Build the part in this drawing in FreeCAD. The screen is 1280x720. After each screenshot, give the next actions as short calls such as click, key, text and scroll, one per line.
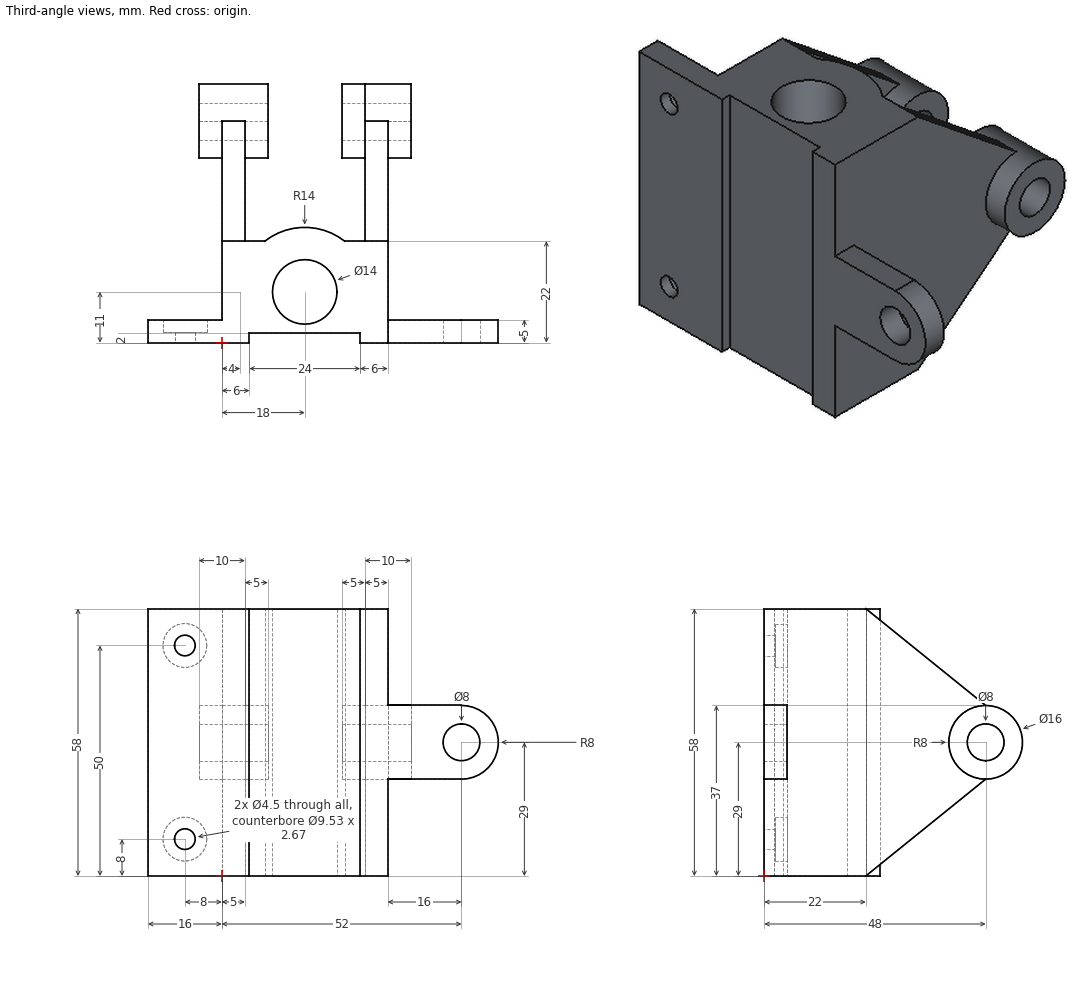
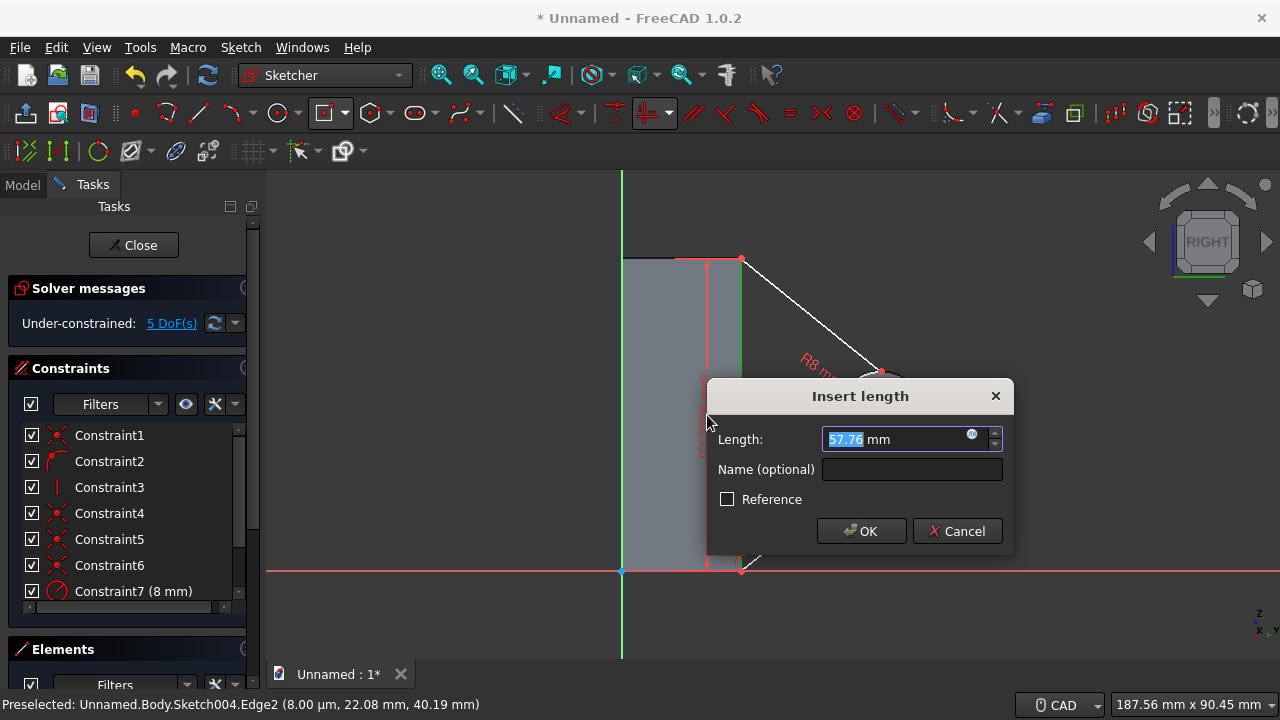
text(58)
key(Return)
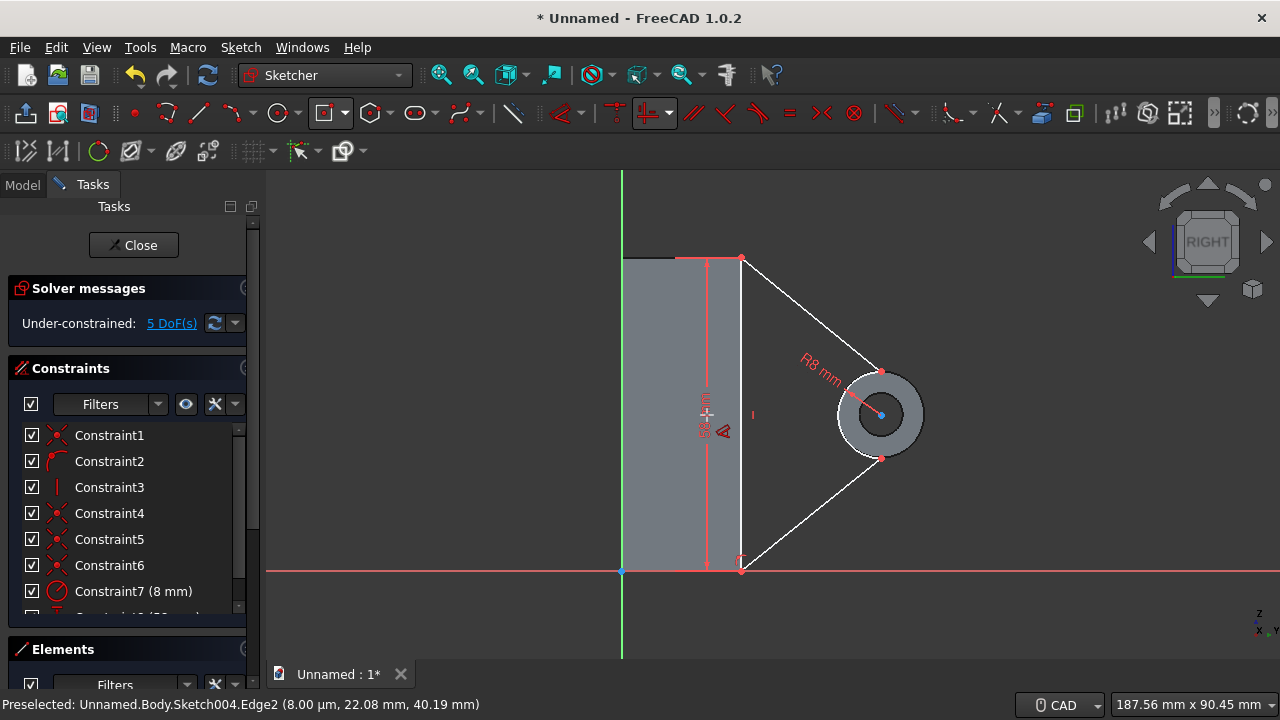
click(881, 372)
click(751, 605)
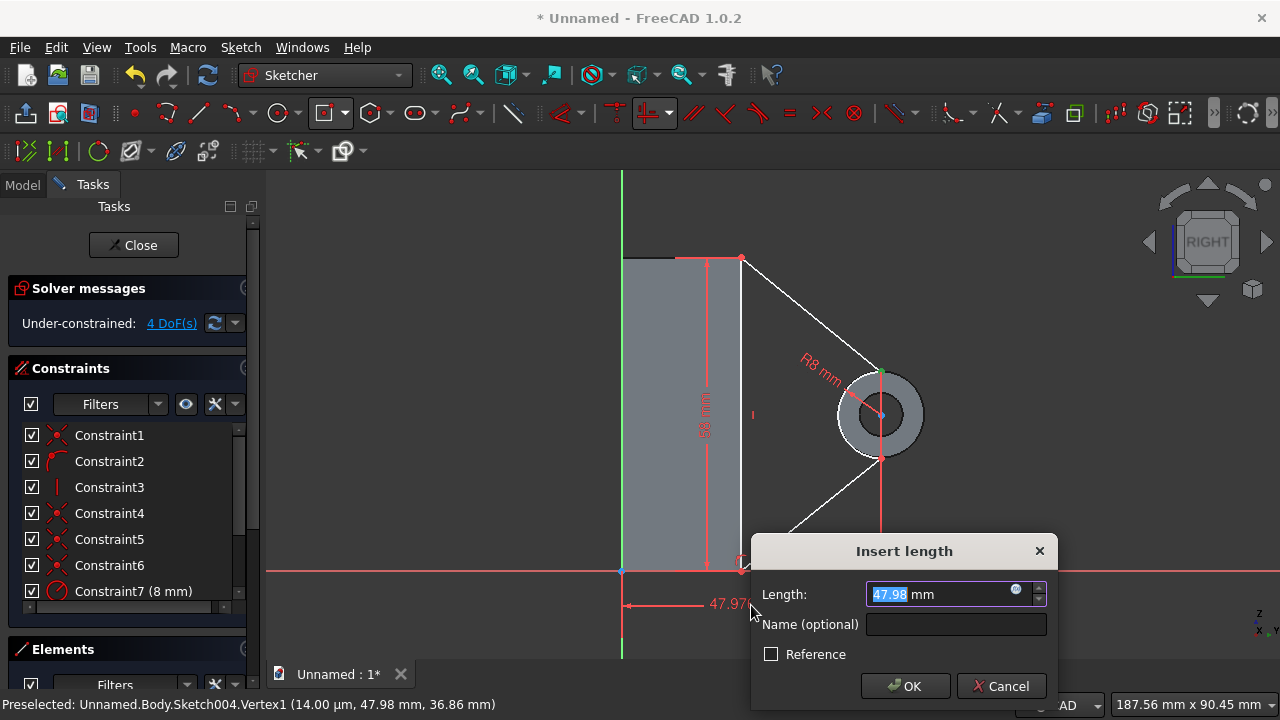
text(48)
key(Return)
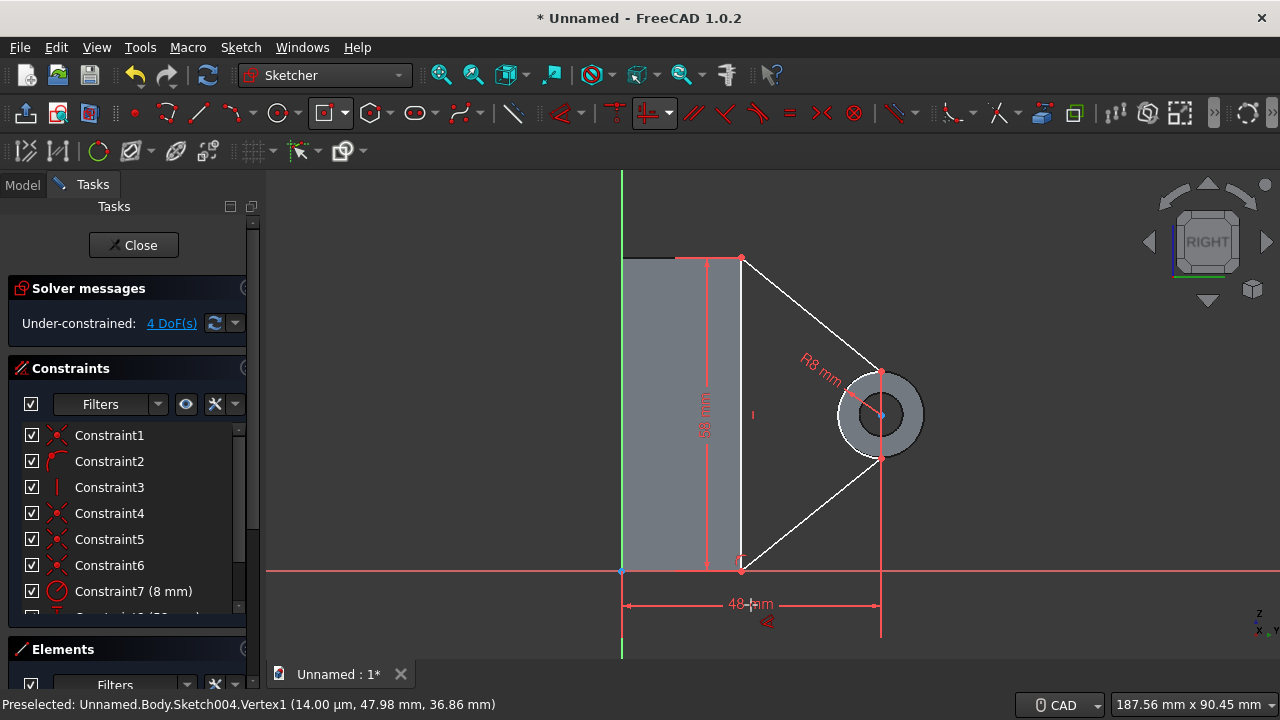
click(881, 372)
click(915, 472)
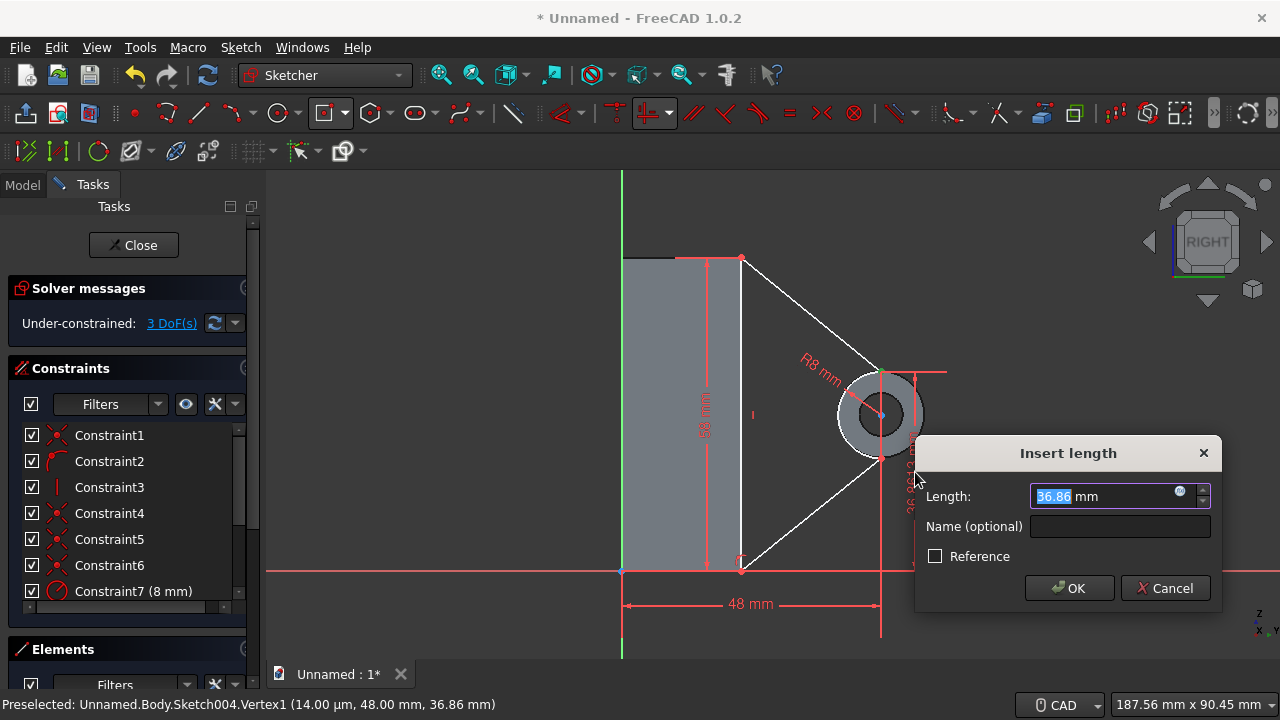
text(37)
key(Return)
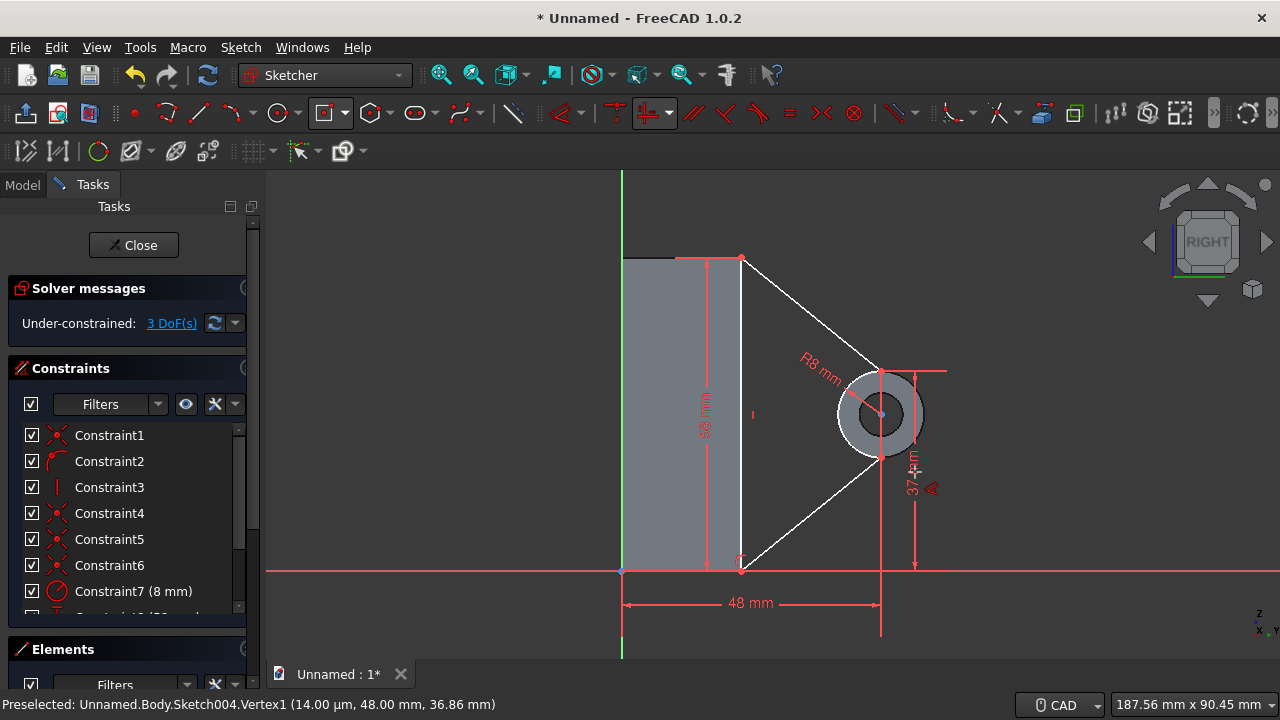
click(741, 258)
click(654, 605)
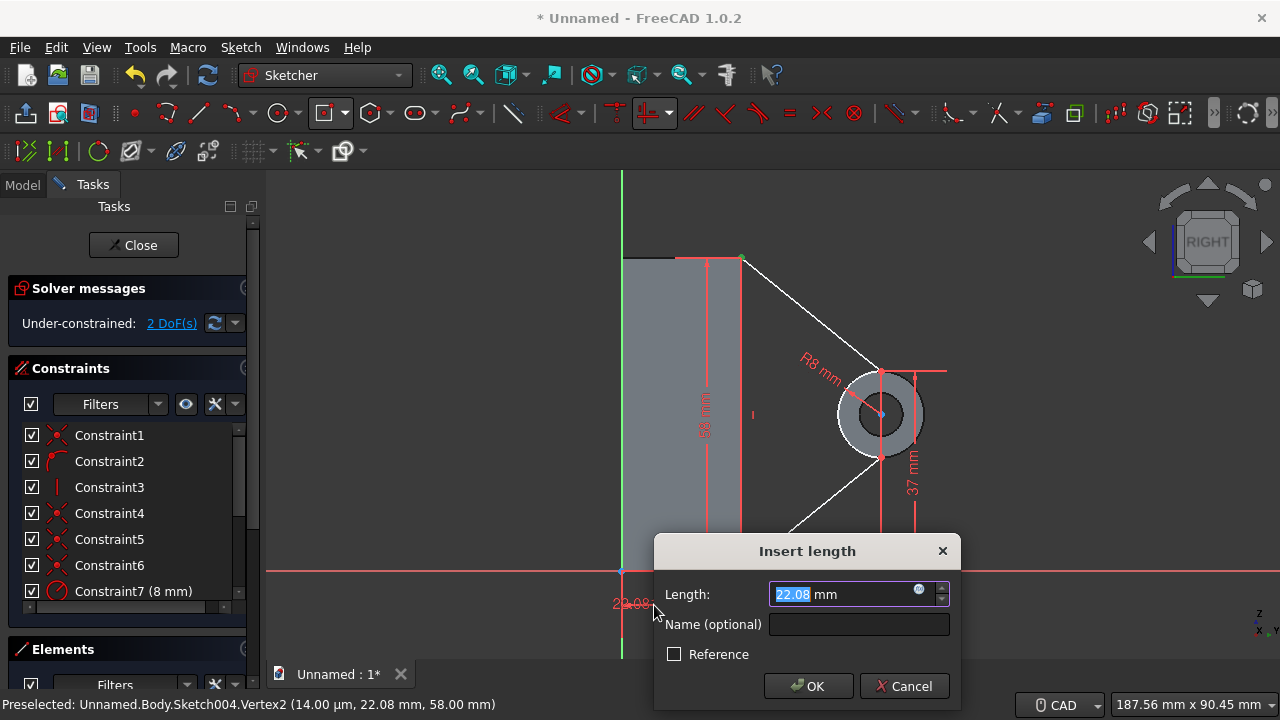
text(22)
key(Return)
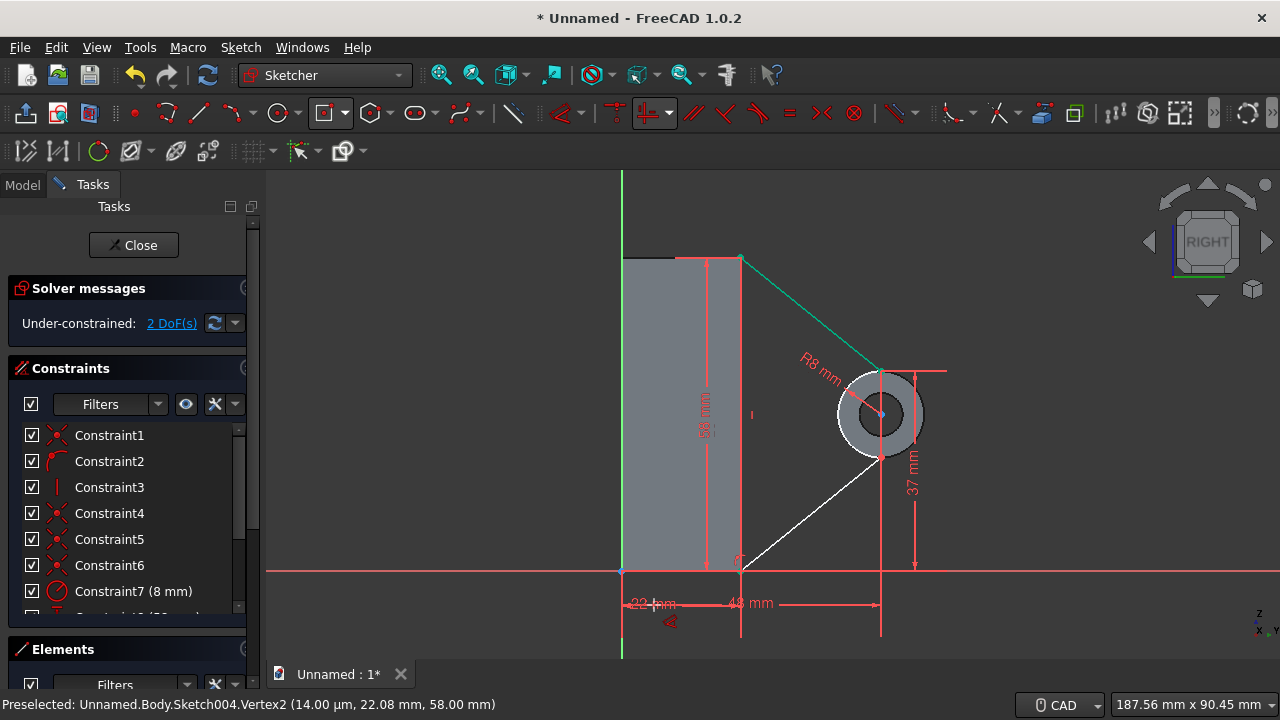
click(881, 458)
click(842, 605)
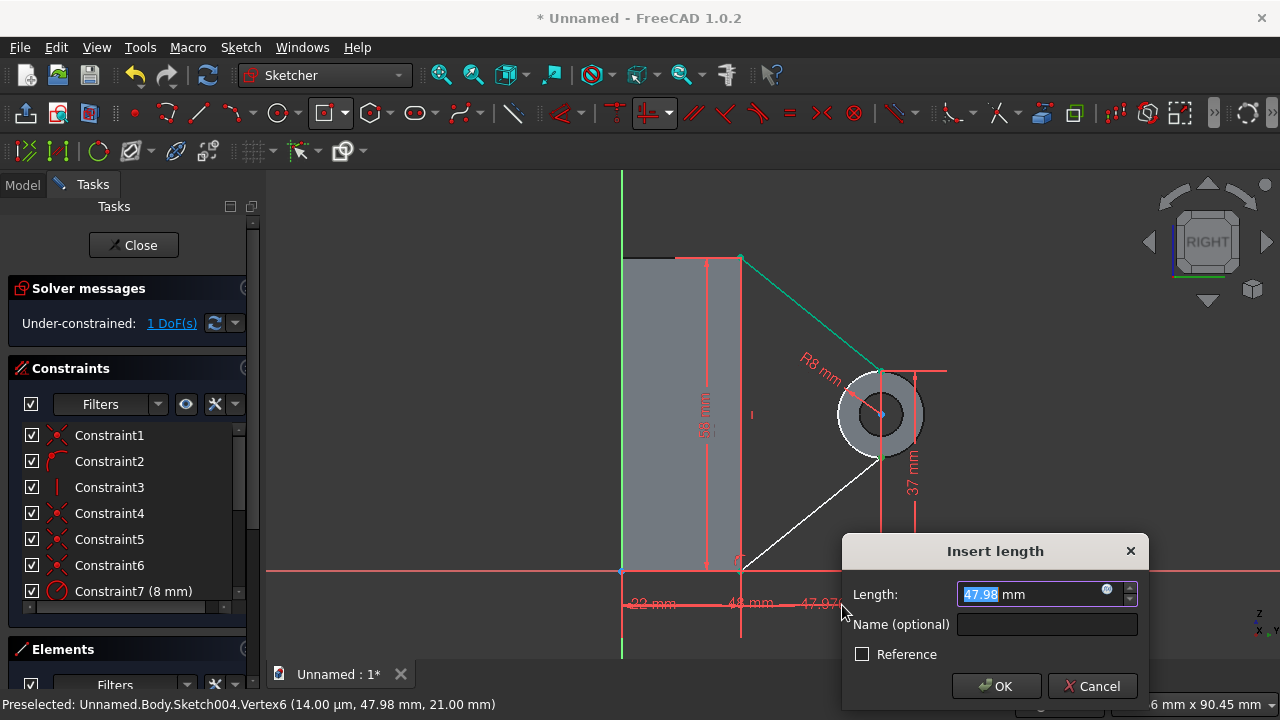
text(48)
key(Return)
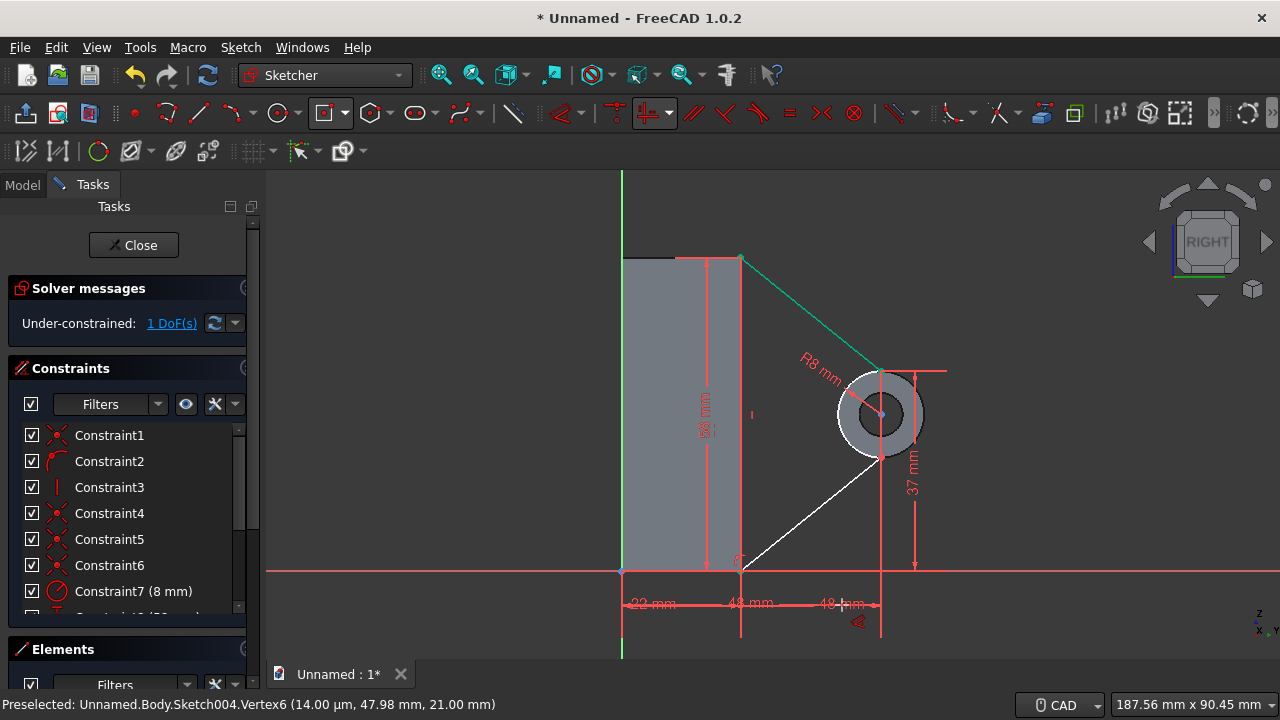
click(882, 414)
click(692, 380)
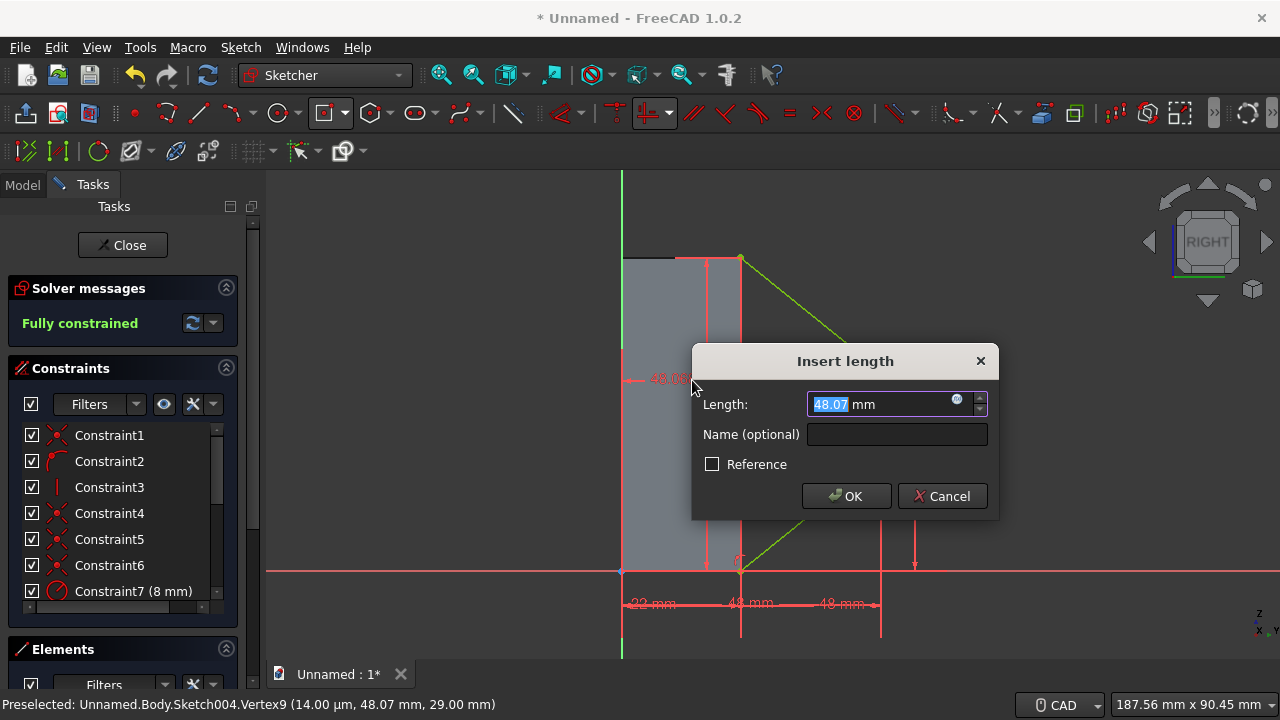
text(48)
key(Return)
key(Escape)